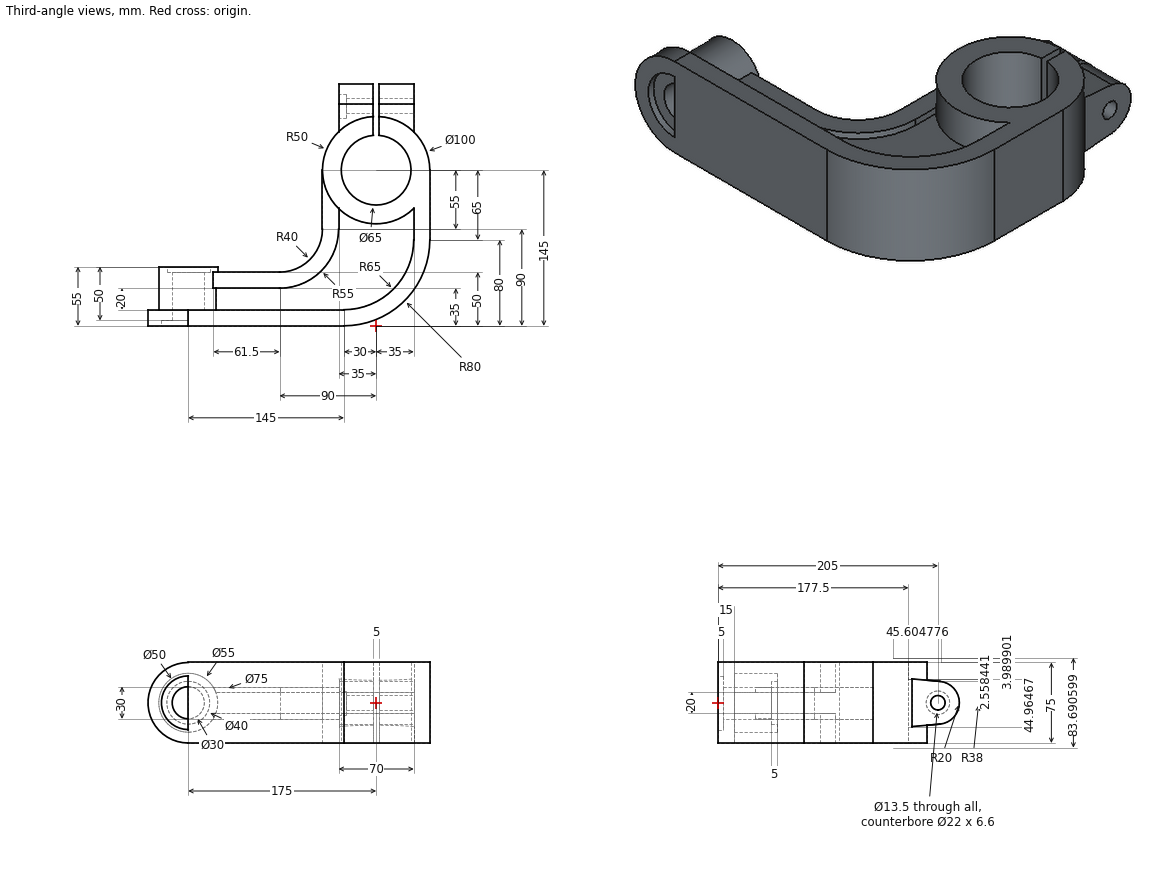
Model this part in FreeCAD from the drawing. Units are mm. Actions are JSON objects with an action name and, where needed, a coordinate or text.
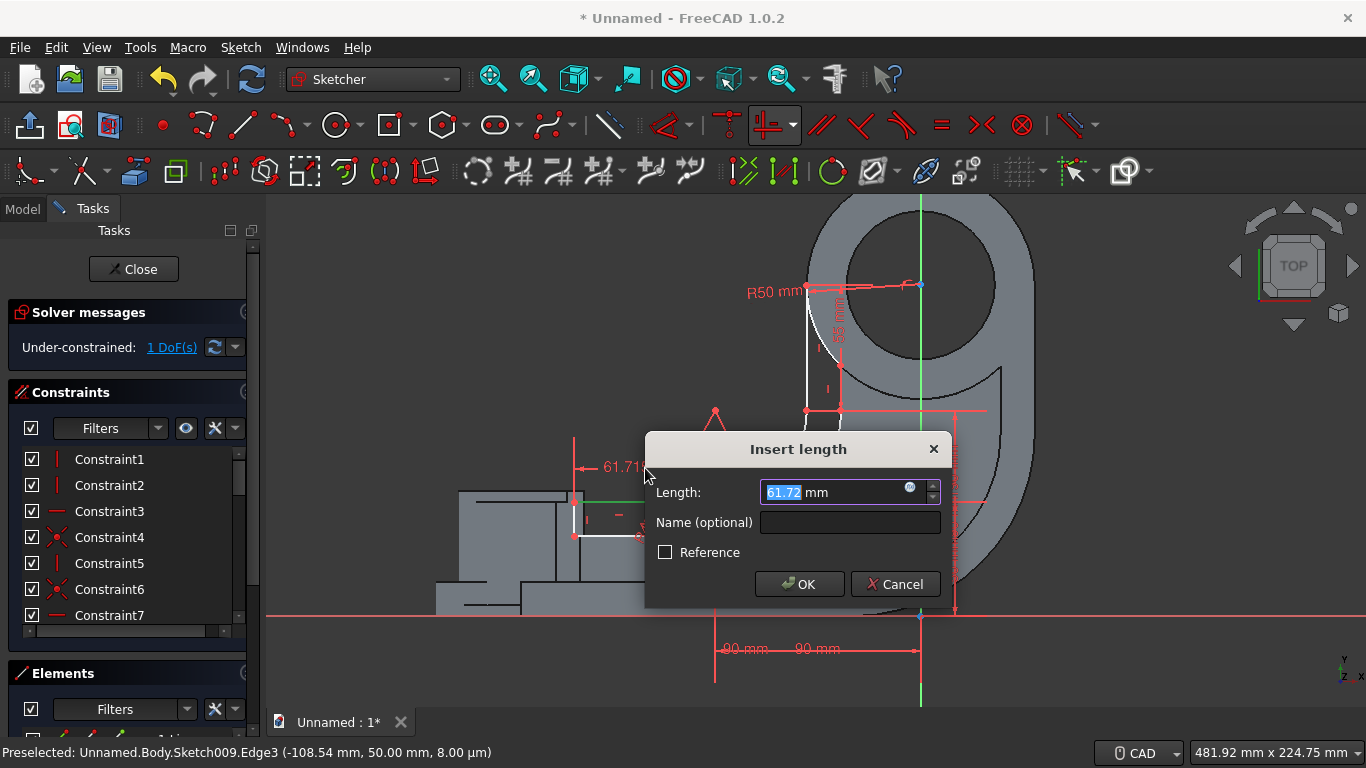
{"action": "type", "text": "61.5"}
{"action": "key", "text": "Return"}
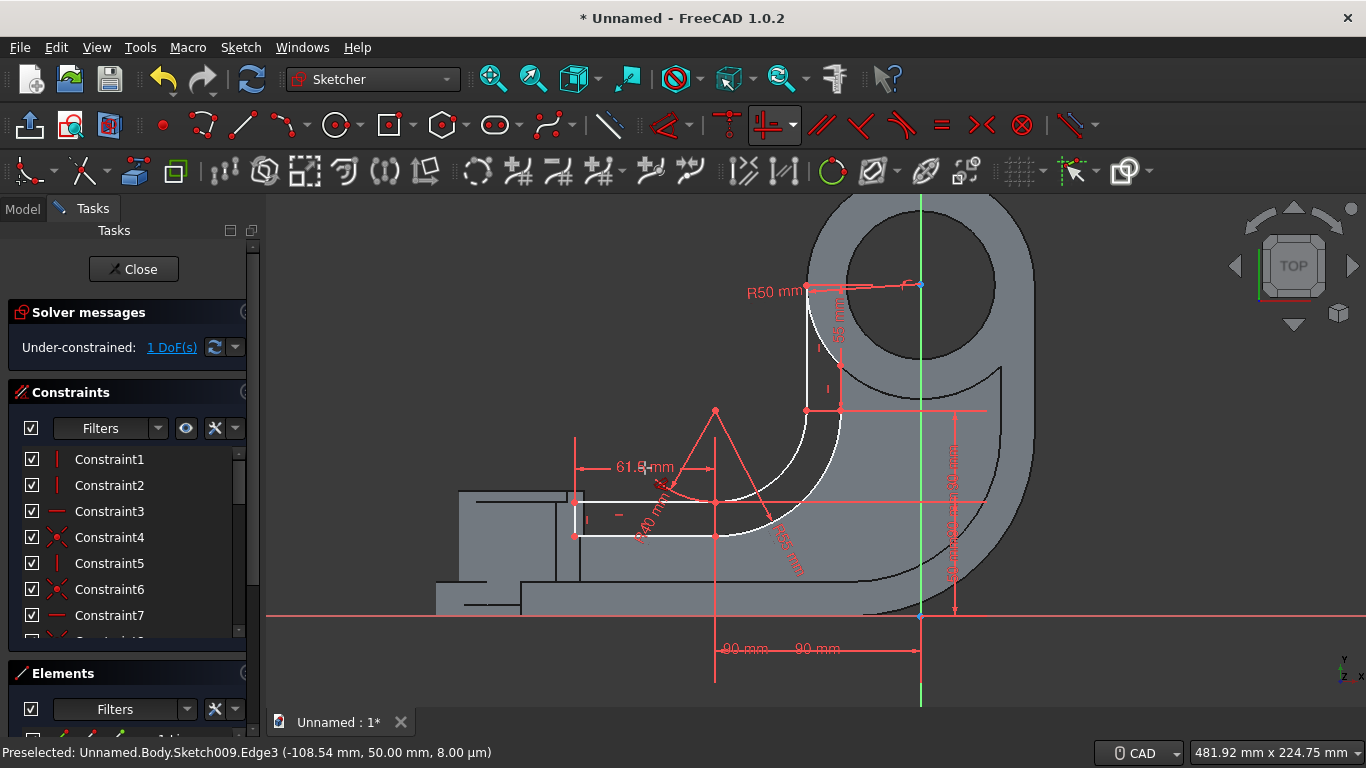
{"action": "left_click", "coordinate": [921, 284]}
{"action": "left_click", "coordinate": [955, 374]}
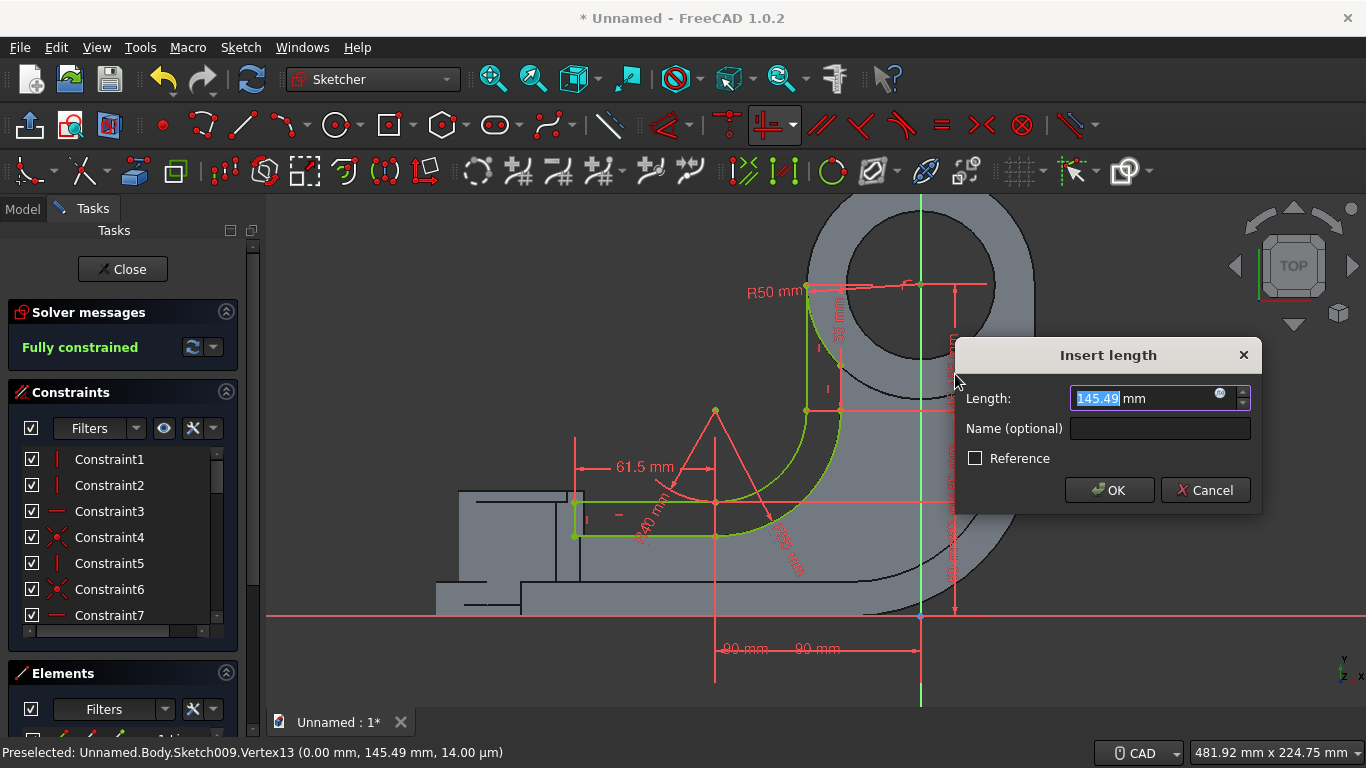
{"action": "type", "text": "145"}
{"action": "key", "text": "Return"}
{"action": "key", "text": "Escape"}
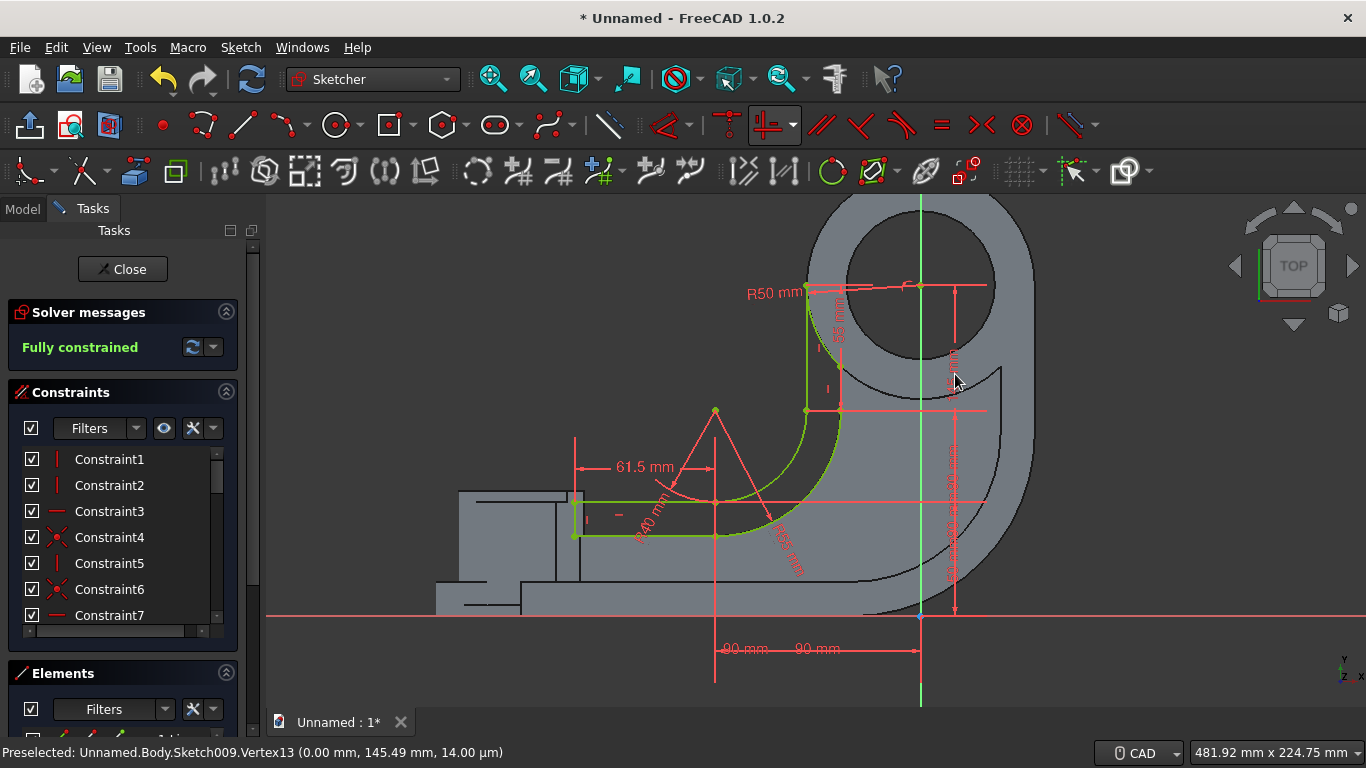
{"action": "left_click", "coordinate": [123, 269]}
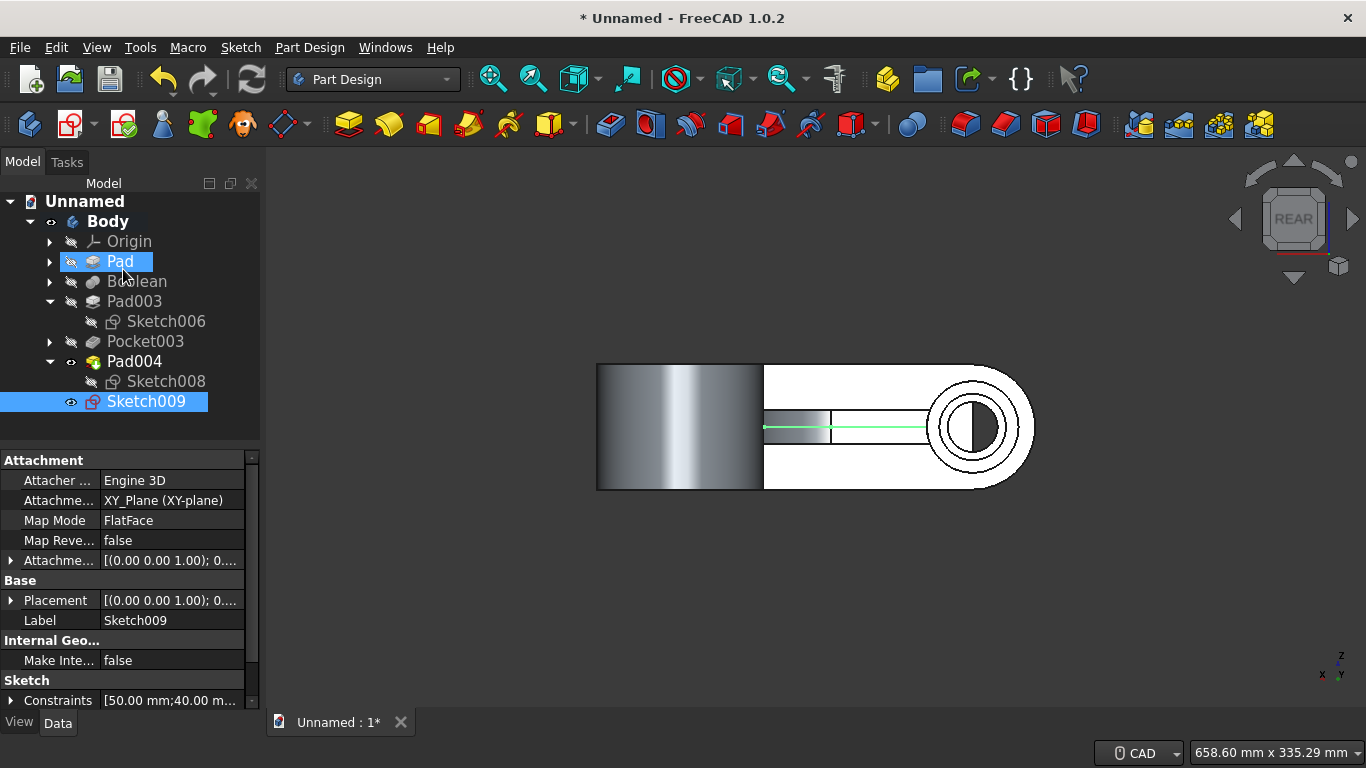
{"action": "left_click", "coordinate": [350, 124]}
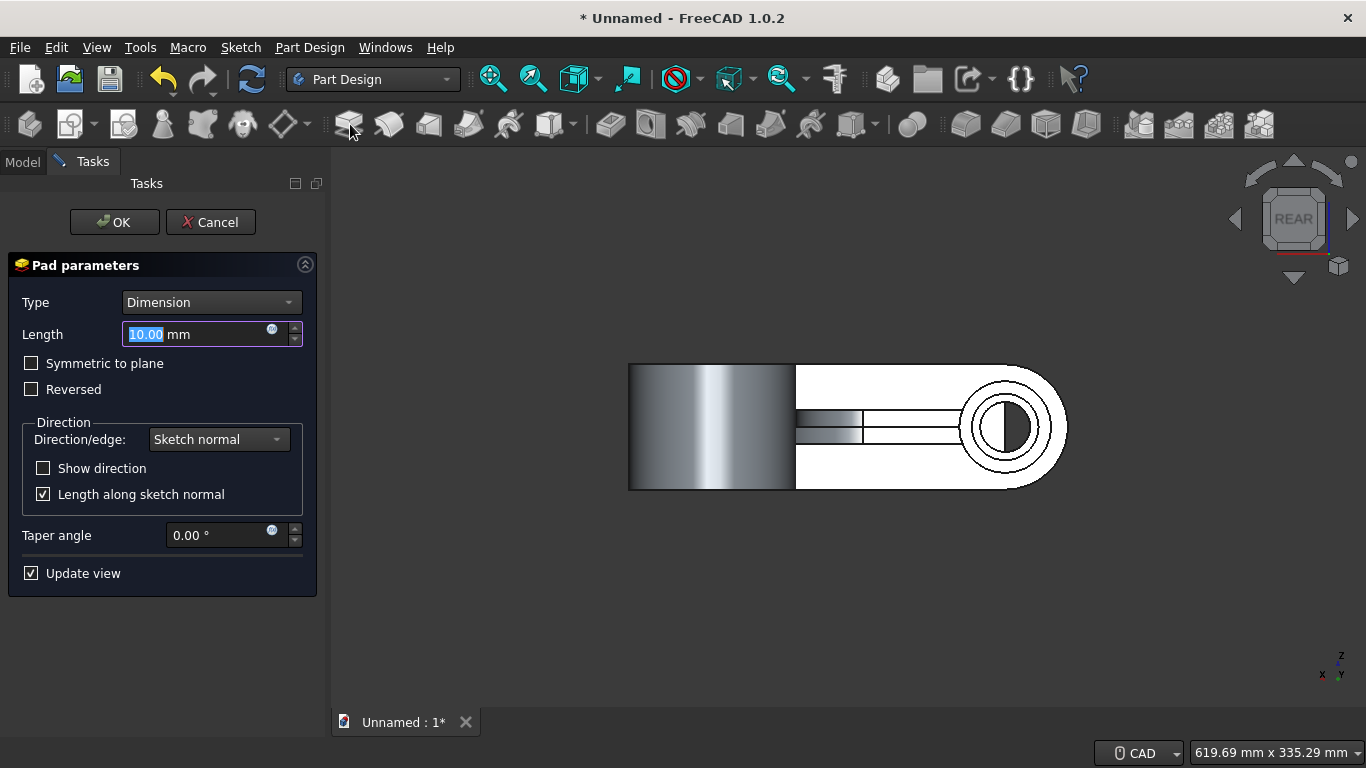
{"action": "type", "text": "30"}
{"action": "key", "text": "Tab"}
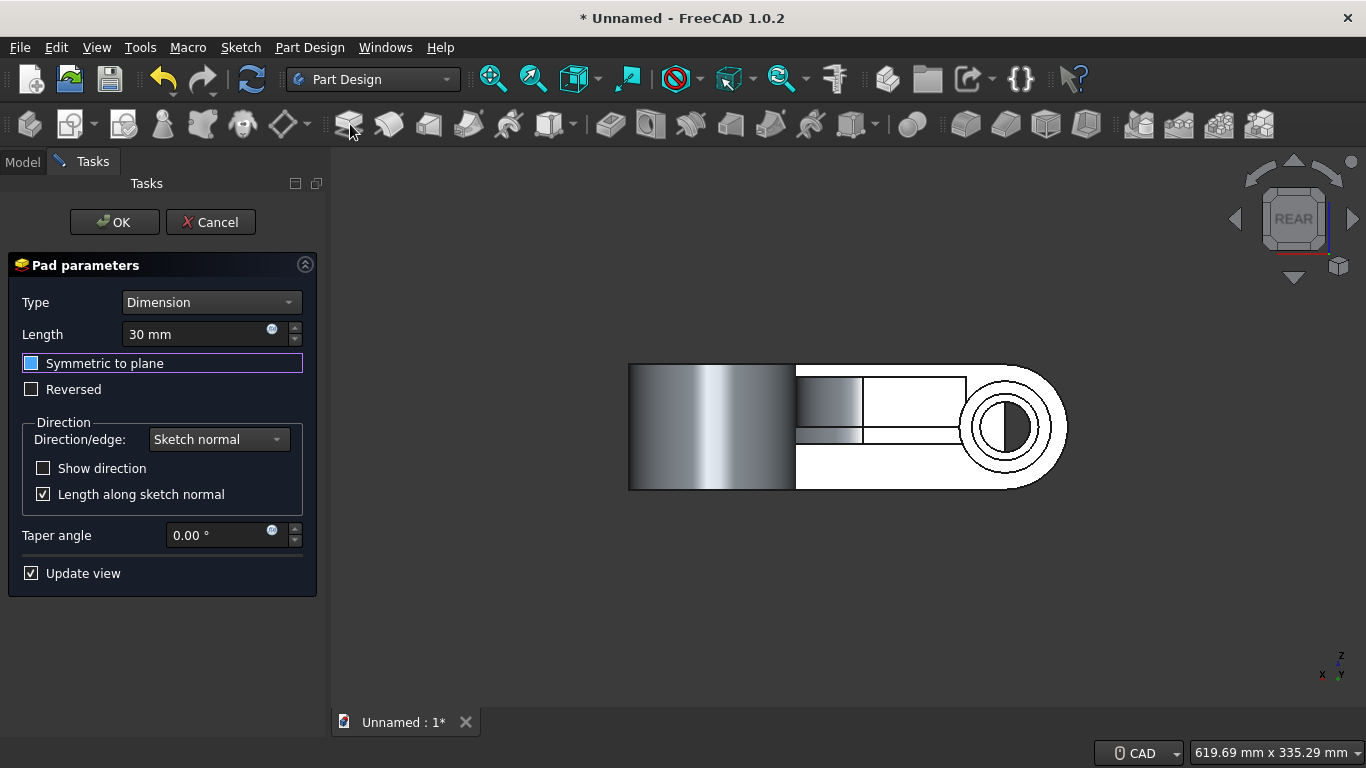
{"action": "left_click", "coordinate": [30, 363]}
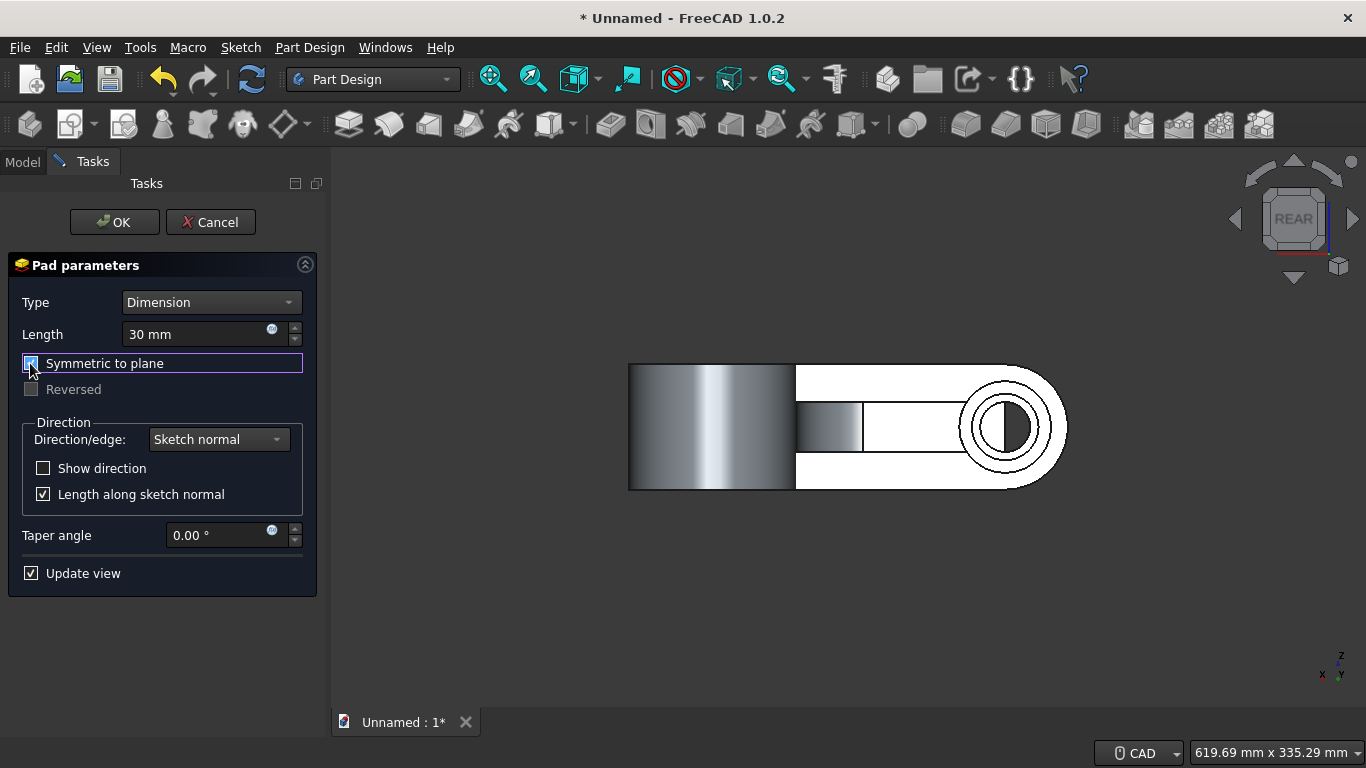
{"action": "left_click", "coordinate": [115, 222]}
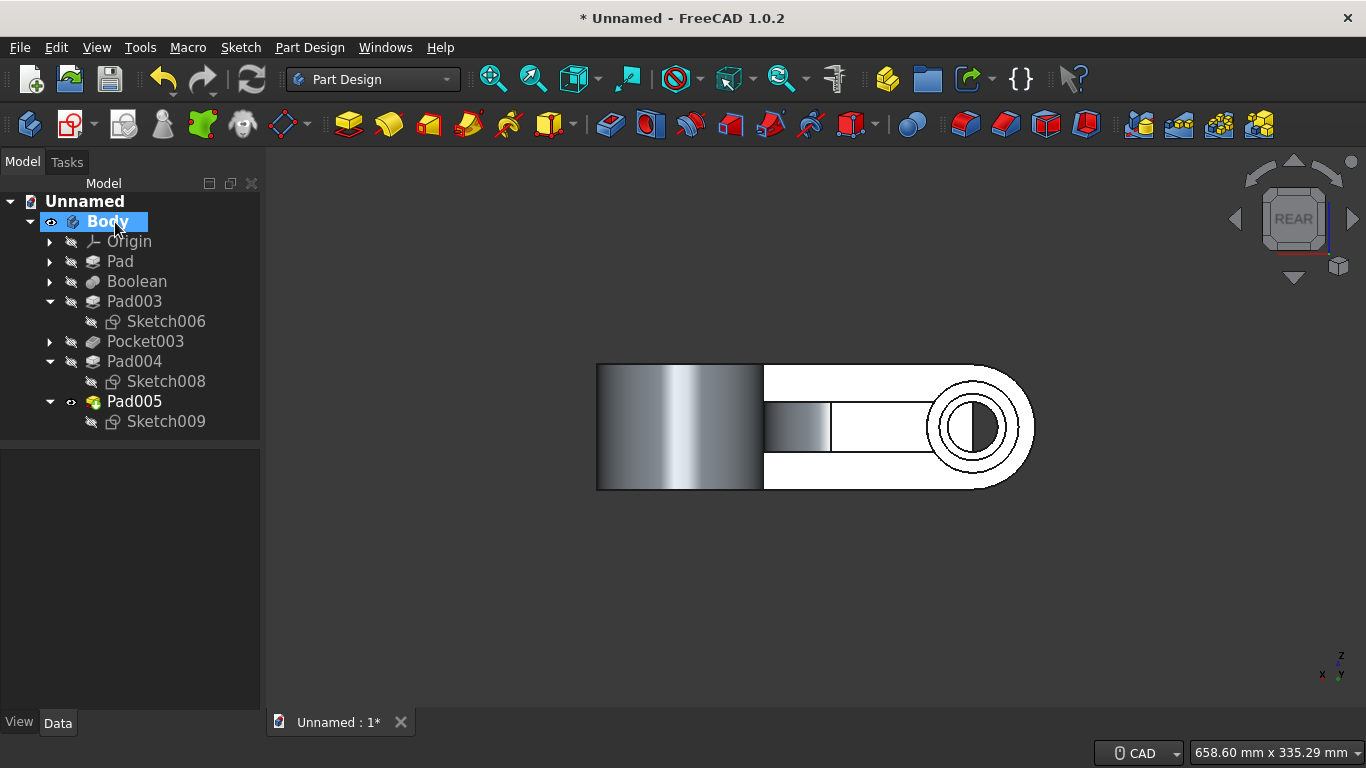
{"action": "left_click", "coordinate": [494, 80]}